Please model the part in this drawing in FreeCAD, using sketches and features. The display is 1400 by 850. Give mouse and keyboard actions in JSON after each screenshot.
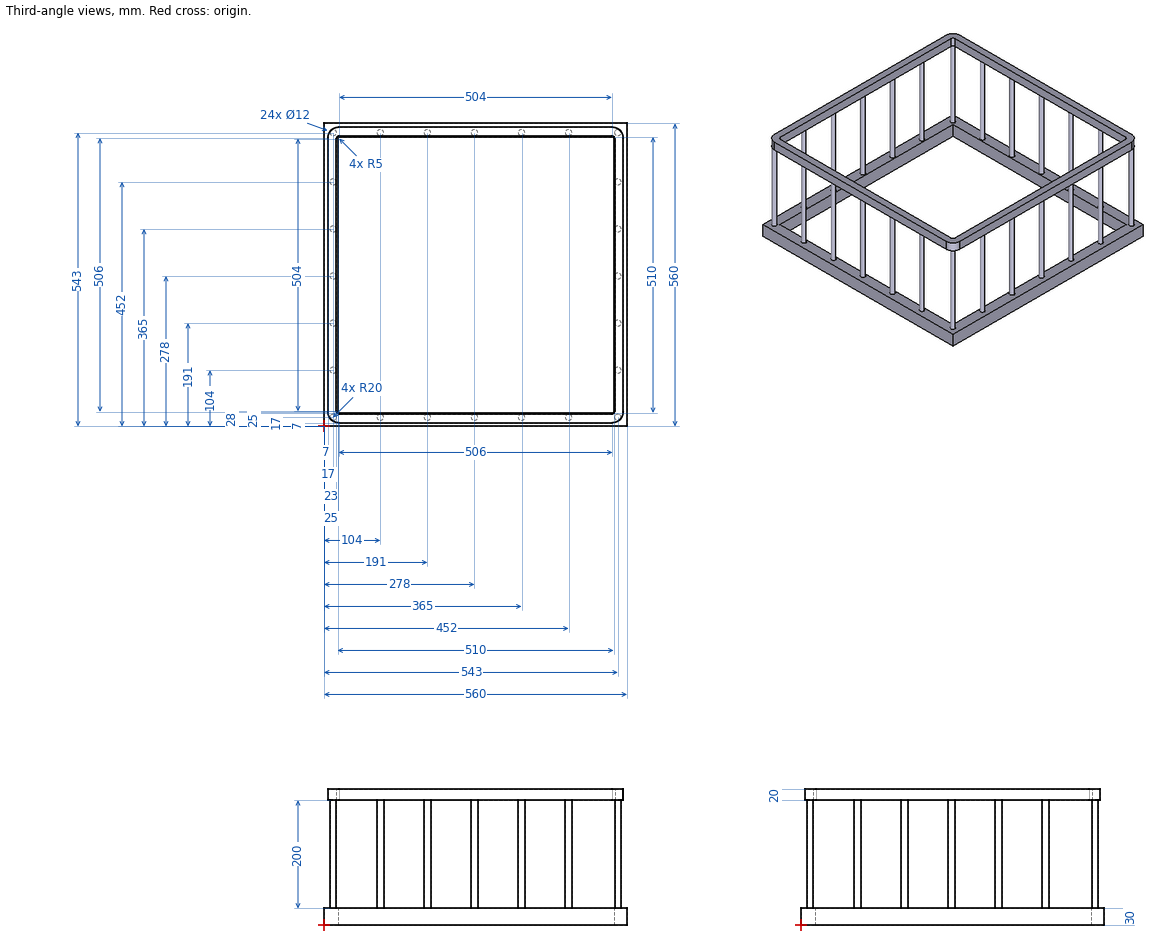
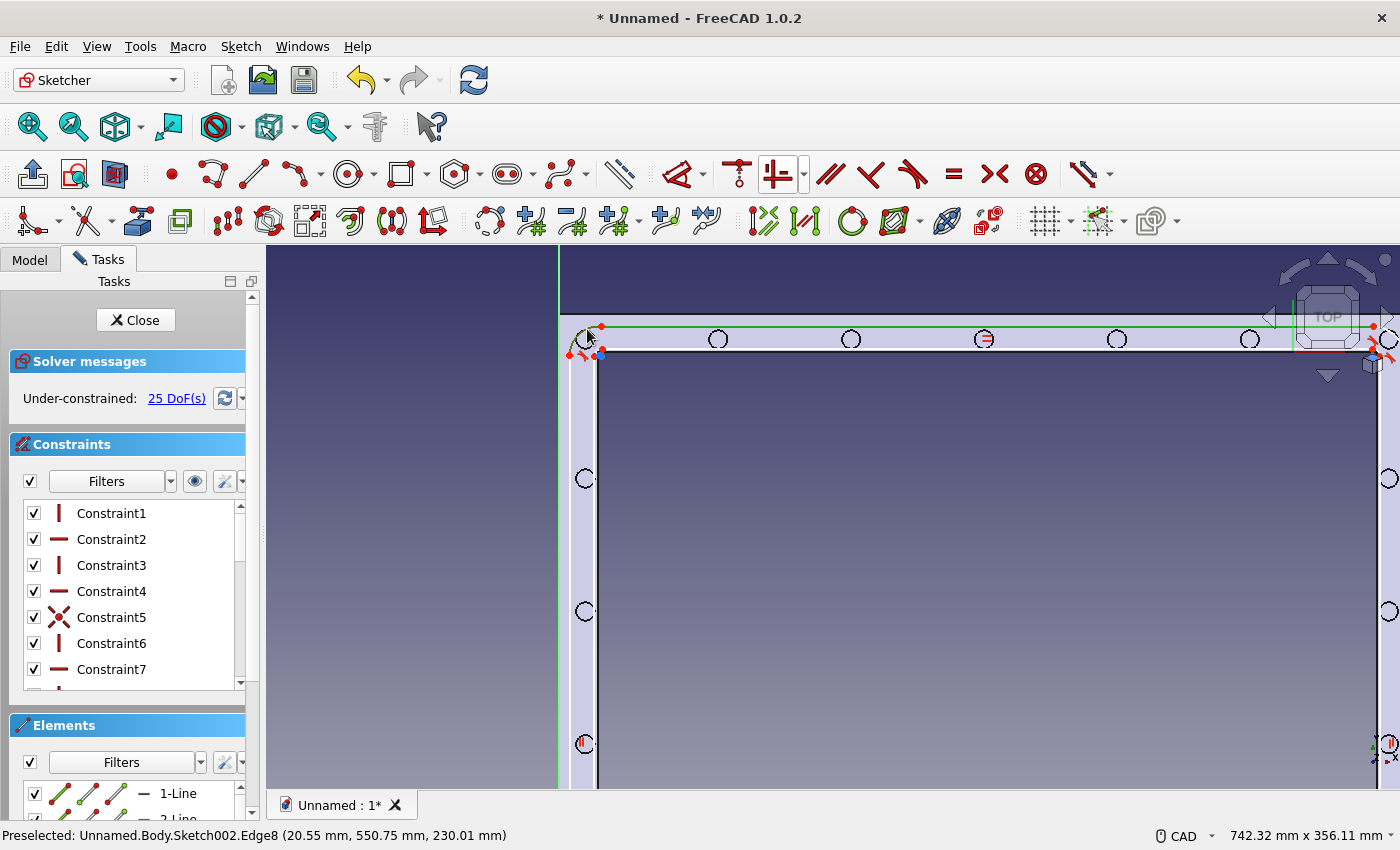
{"action": "left_click", "coordinate": [913, 174]}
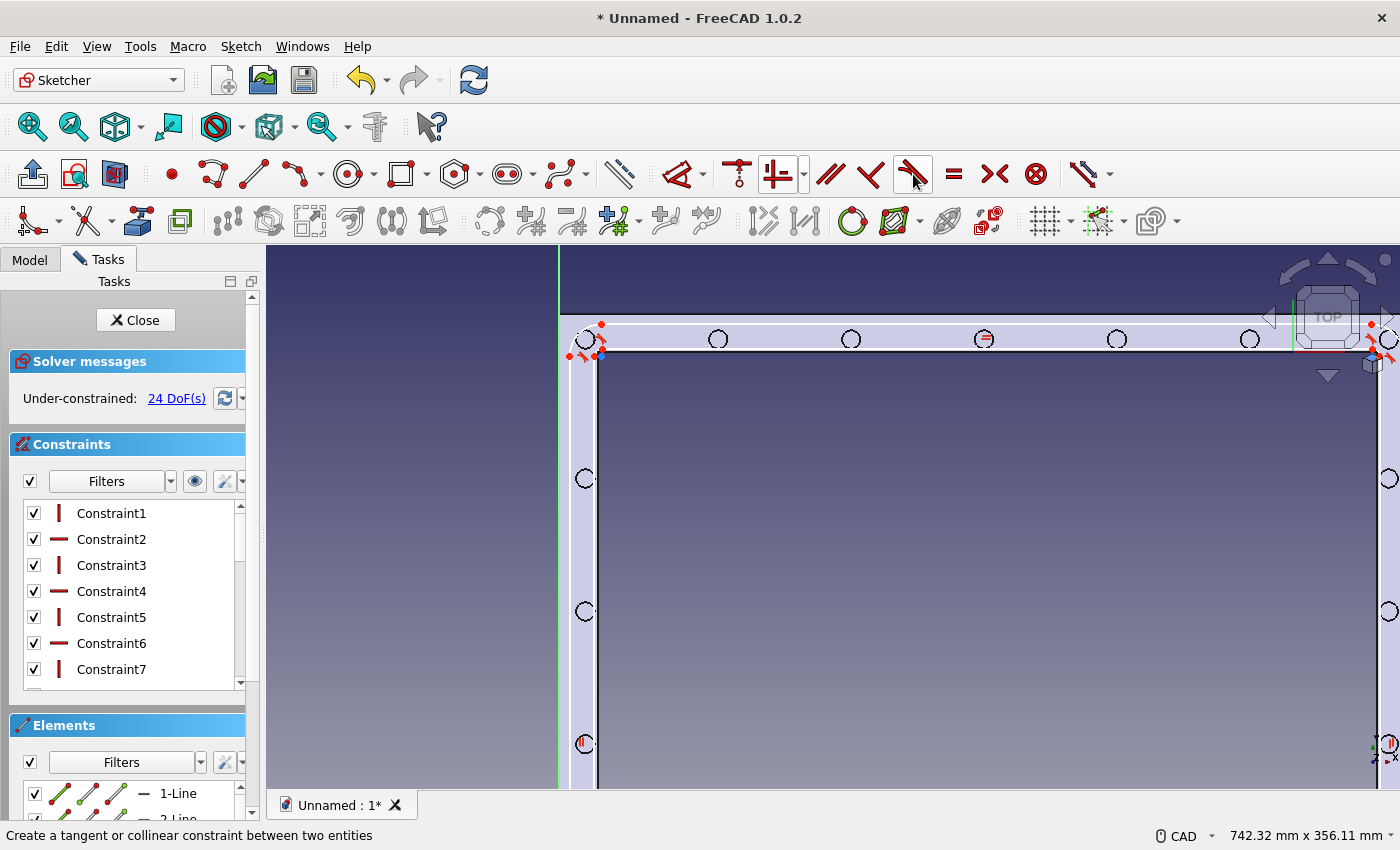
{"action": "left_click", "coordinate": [594, 588]}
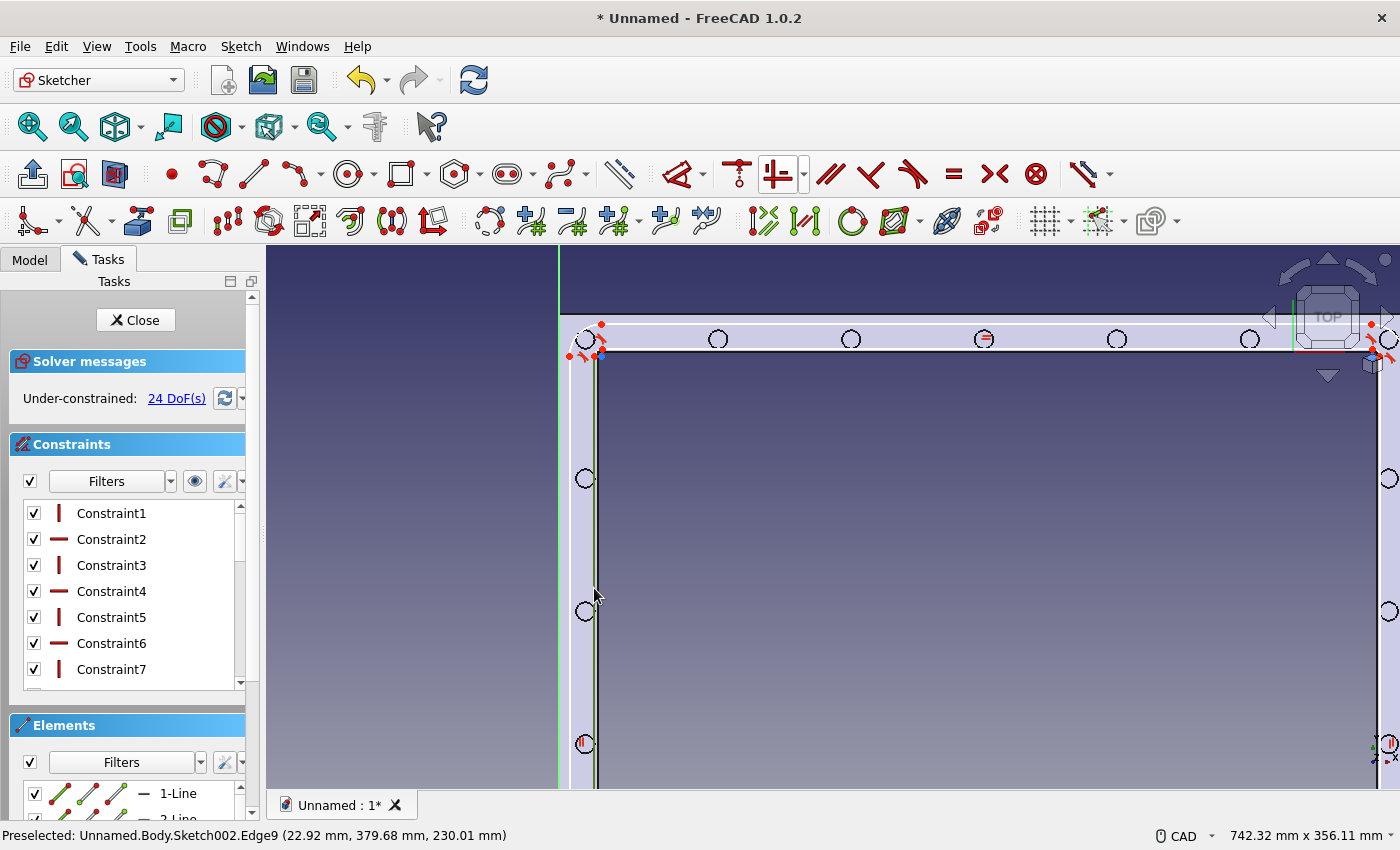
{"action": "scroll", "coordinate": [597, 351], "scroll_direction": "up", "scroll_amount": 5}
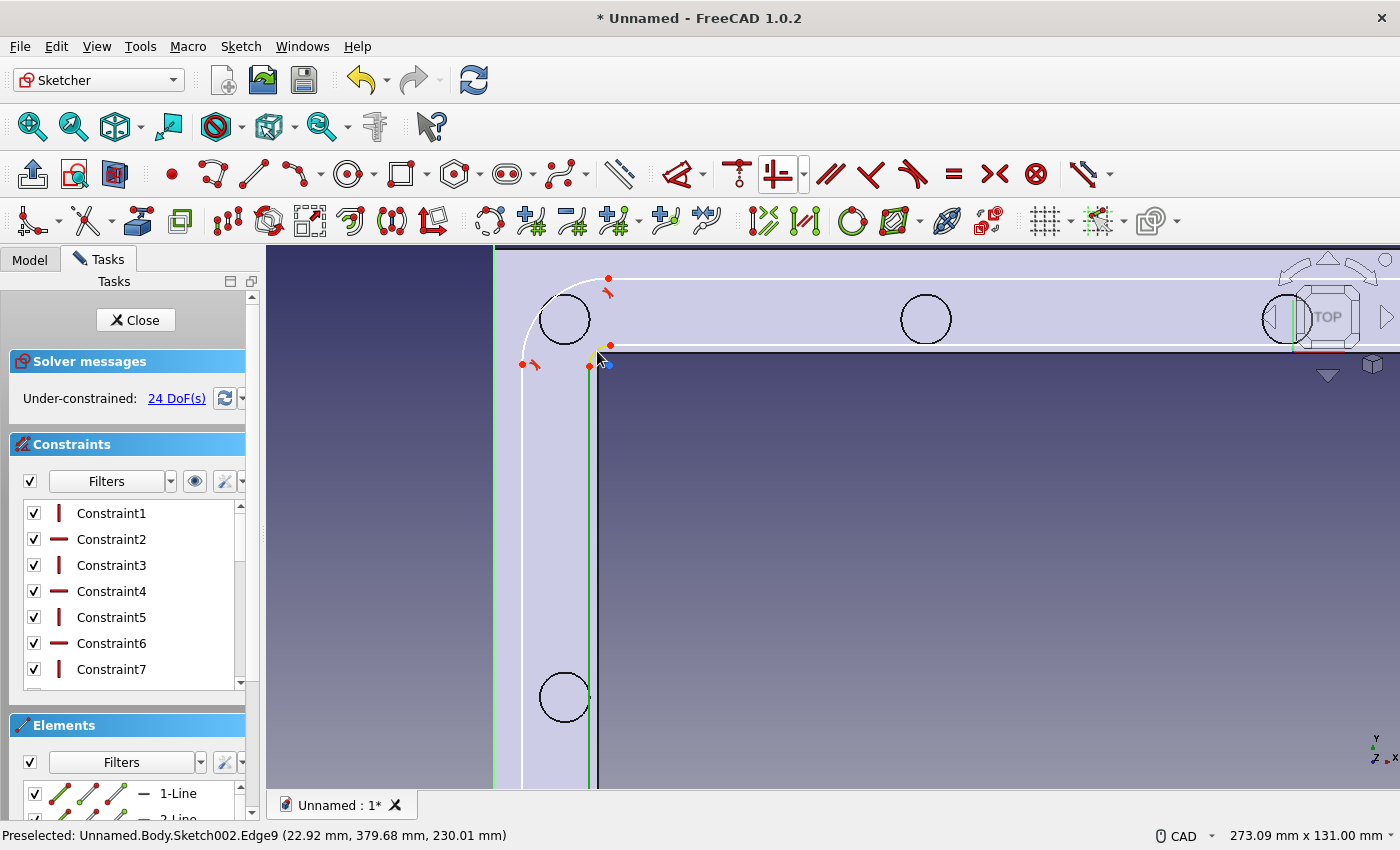
{"action": "left_click", "coordinate": [595, 351]}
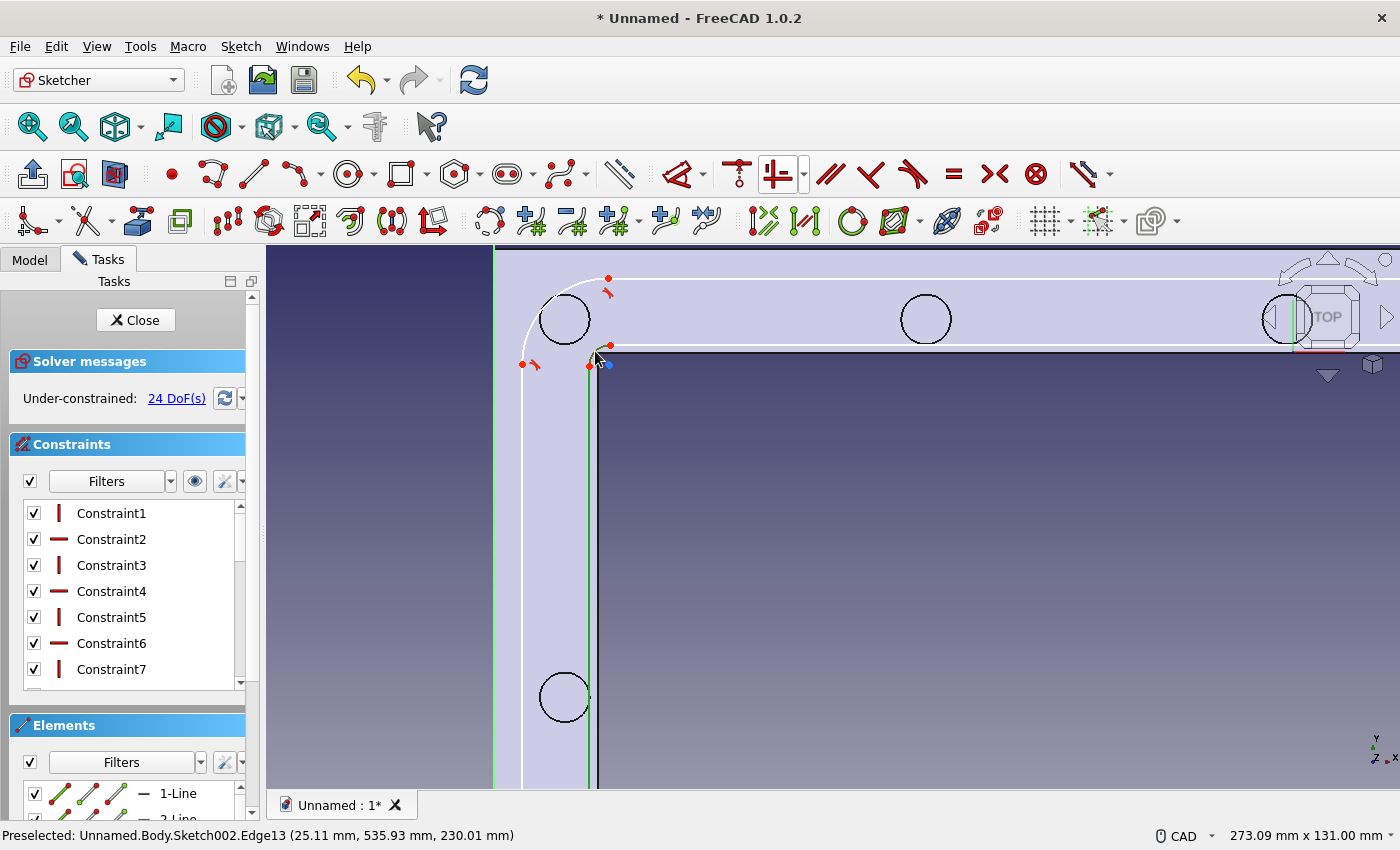
{"action": "left_click", "coordinate": [913, 174]}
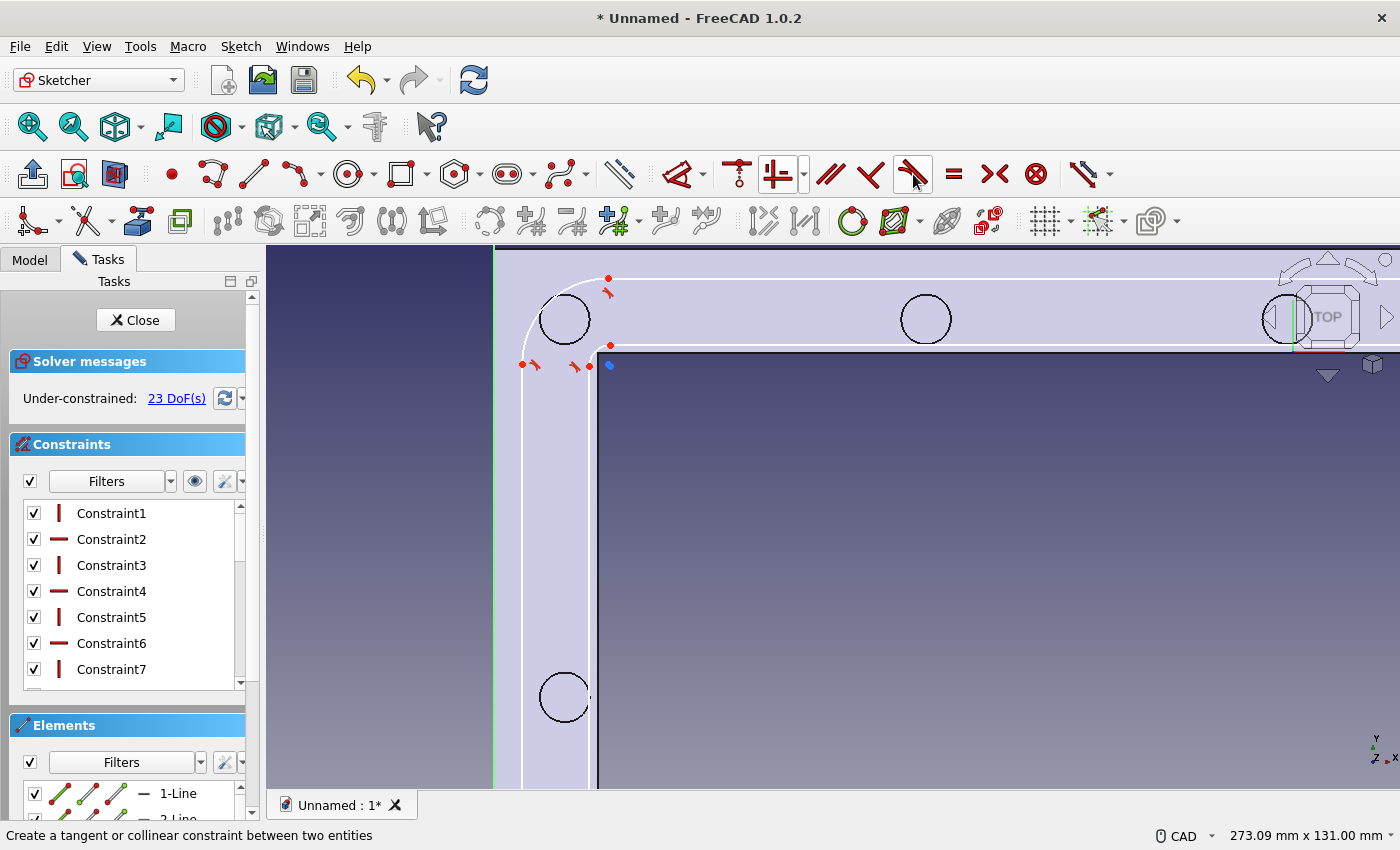
{"action": "scroll", "coordinate": [591, 337], "scroll_direction": "down", "scroll_amount": 9}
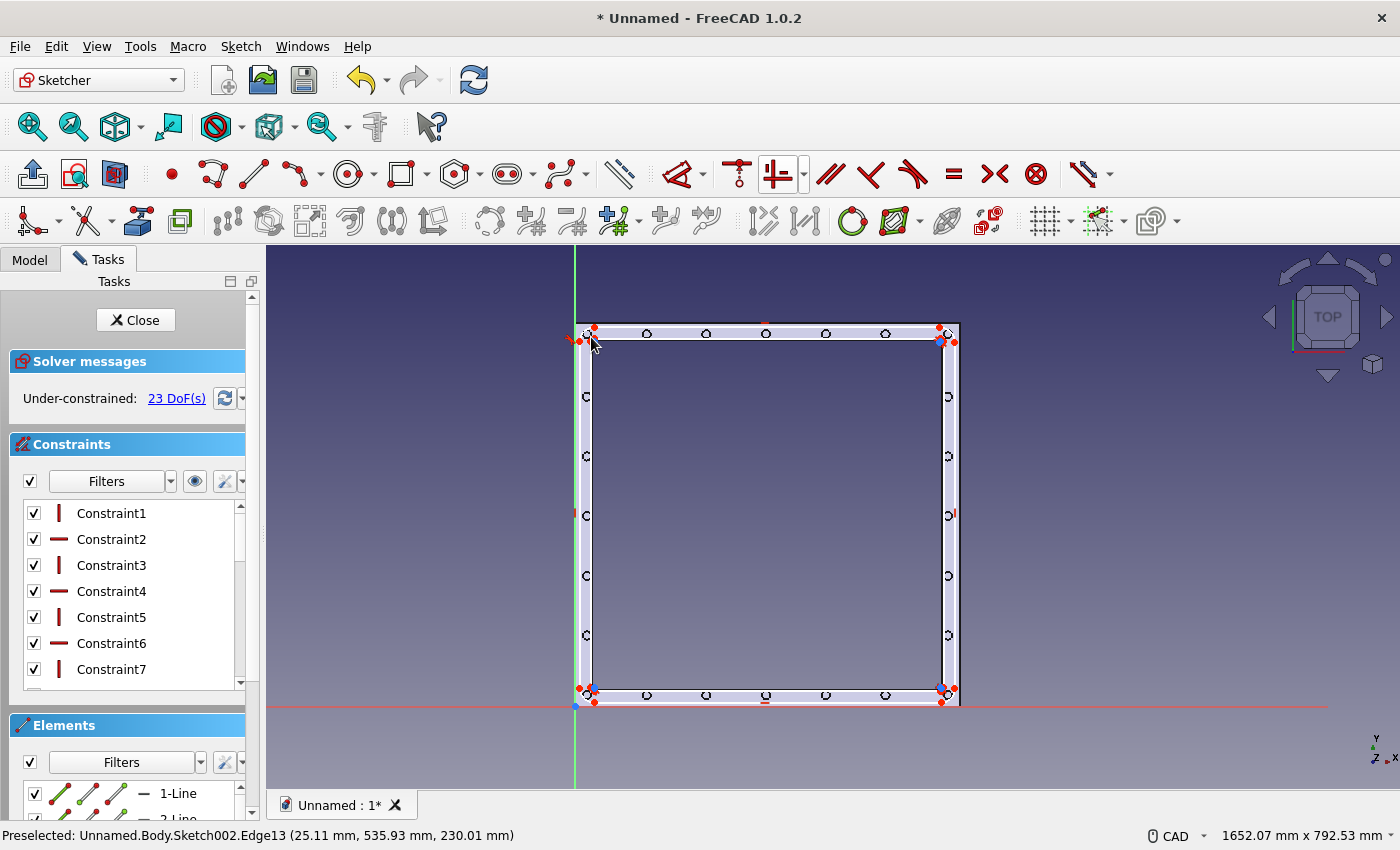
{"action": "scroll", "coordinate": [591, 584], "scroll_direction": "up", "scroll_amount": 2}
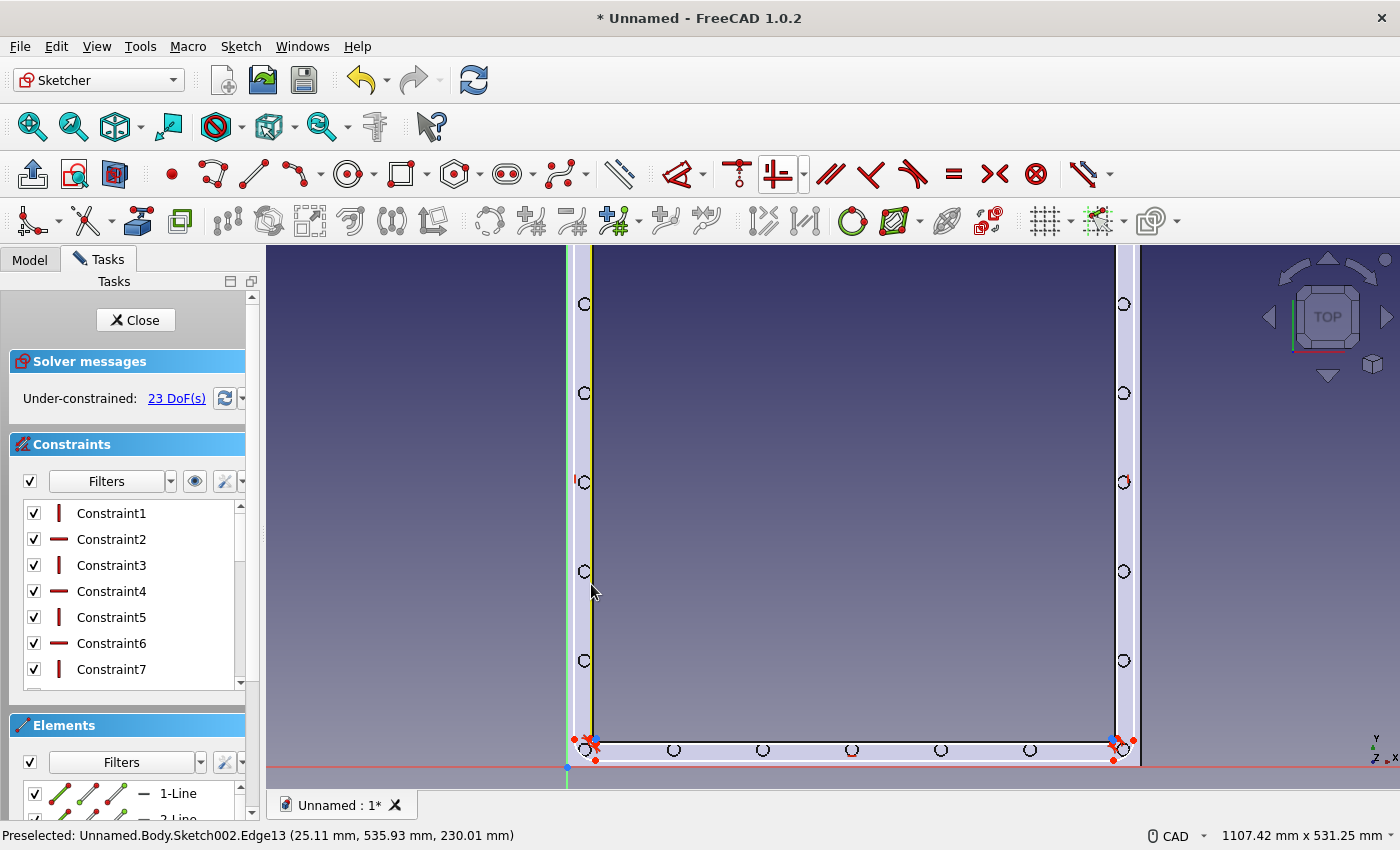
{"action": "left_click", "coordinate": [591, 584]}